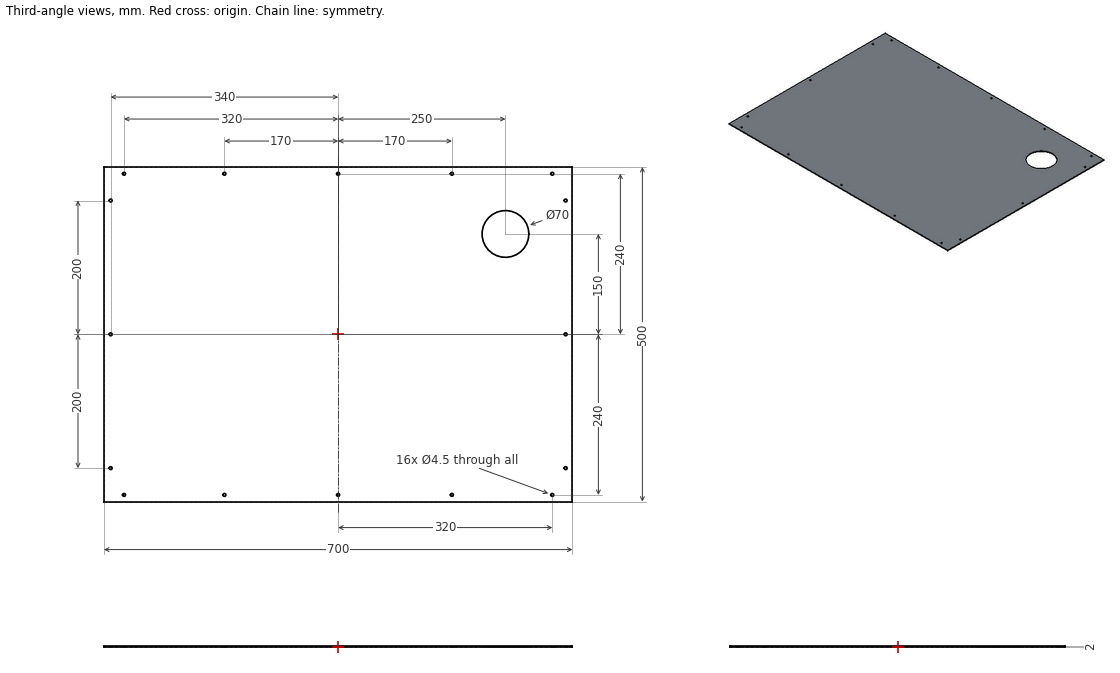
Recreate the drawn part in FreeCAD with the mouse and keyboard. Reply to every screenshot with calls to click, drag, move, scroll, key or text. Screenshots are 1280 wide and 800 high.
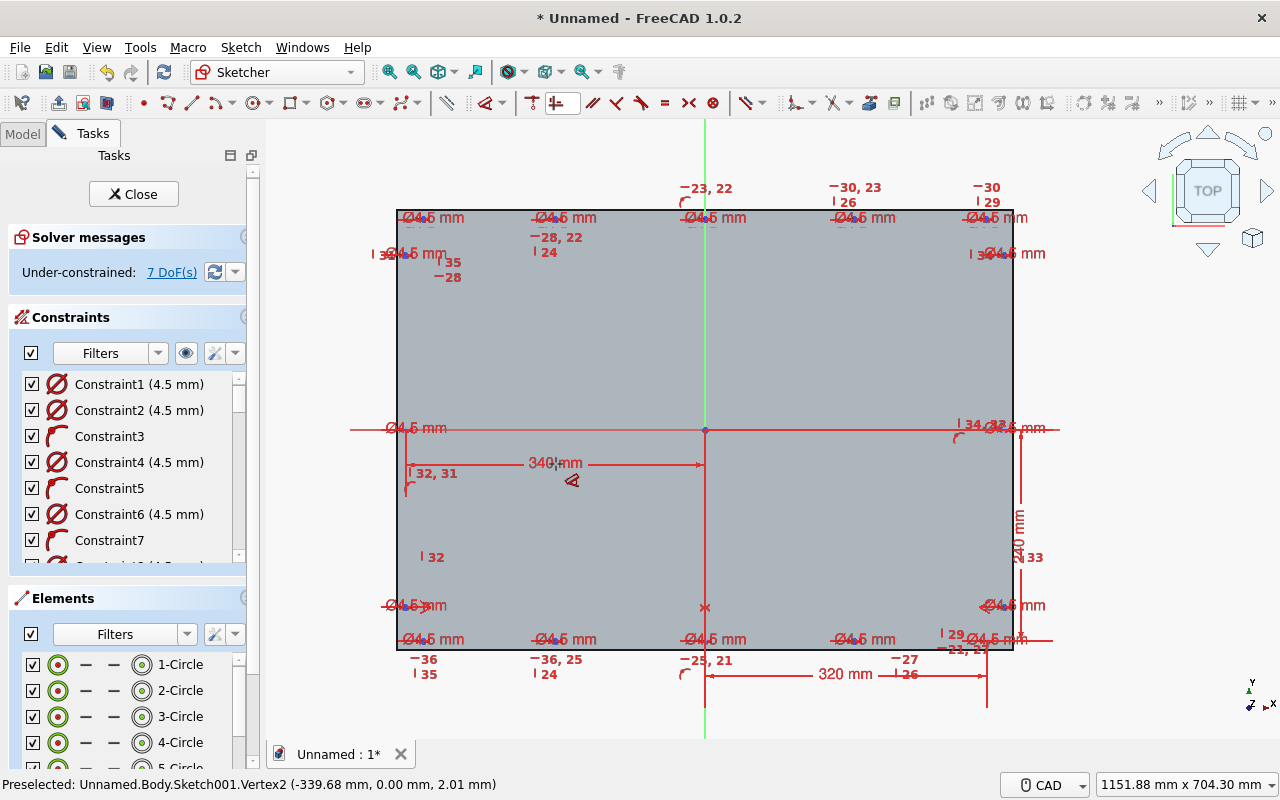
click(705, 220)
click(739, 325)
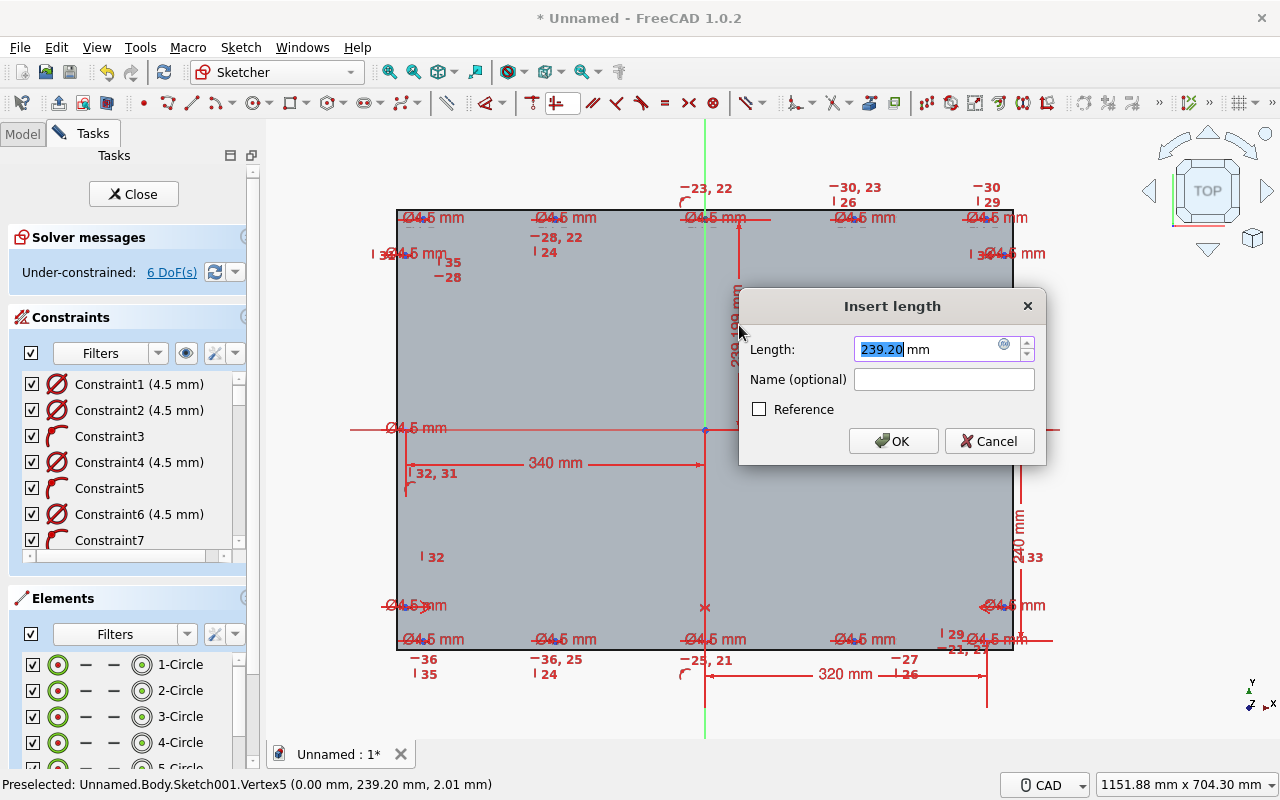
text(240)
key(Return)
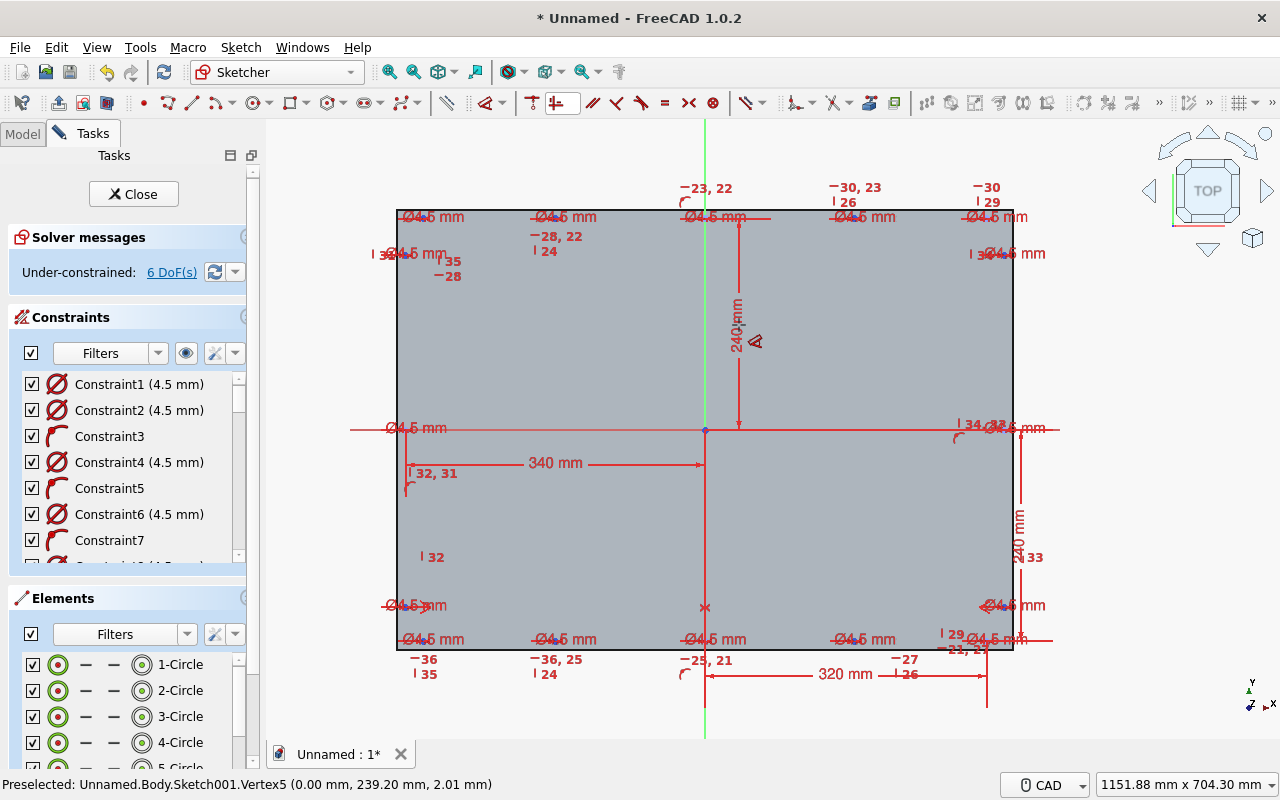
click(556, 219)
click(630, 185)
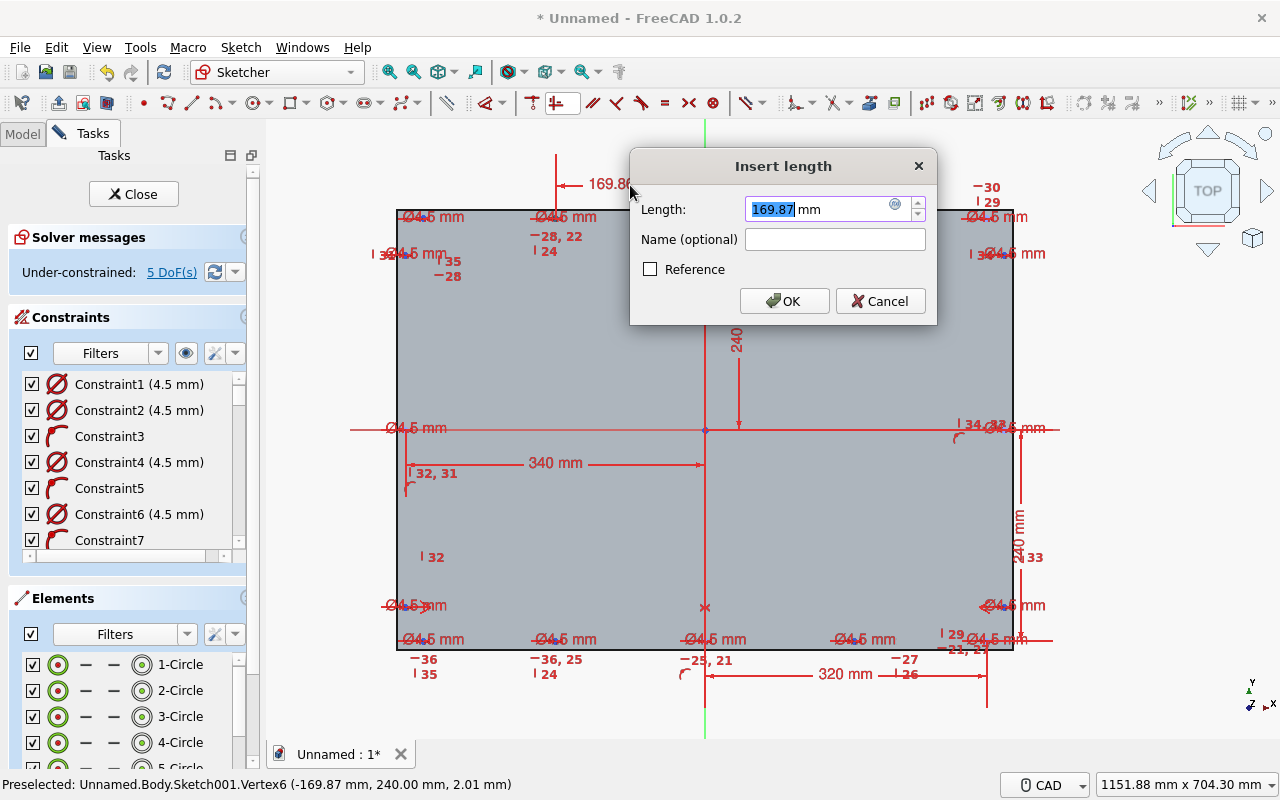
text(170)
key(Return)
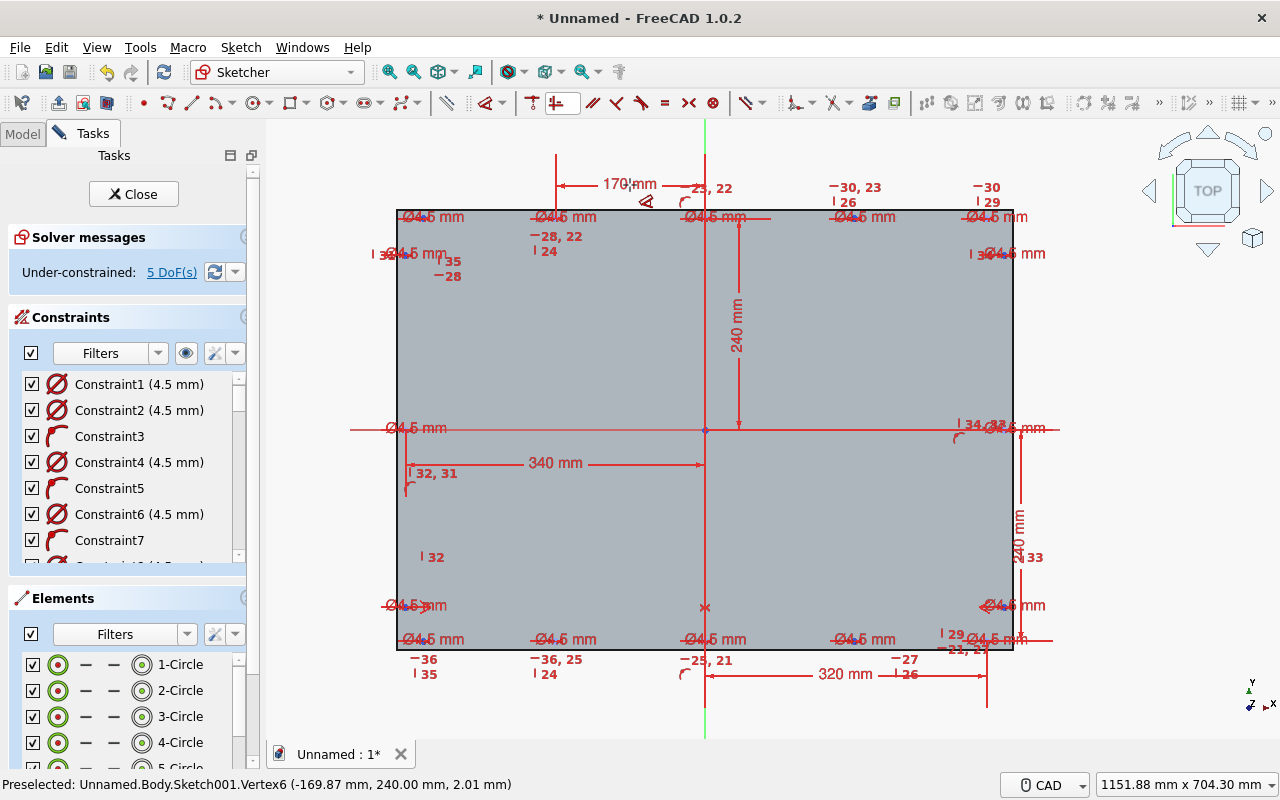
click(855, 219)
click(780, 185)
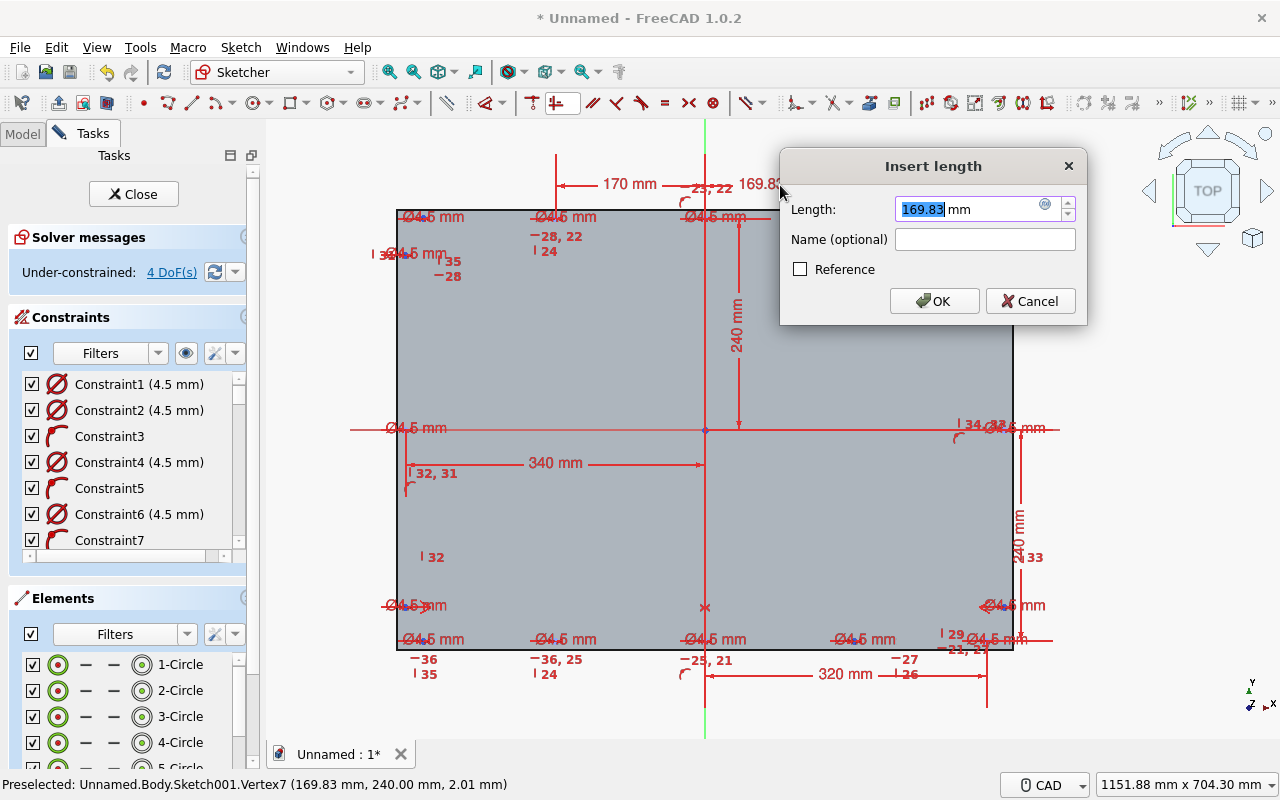
text(170)
key(Return)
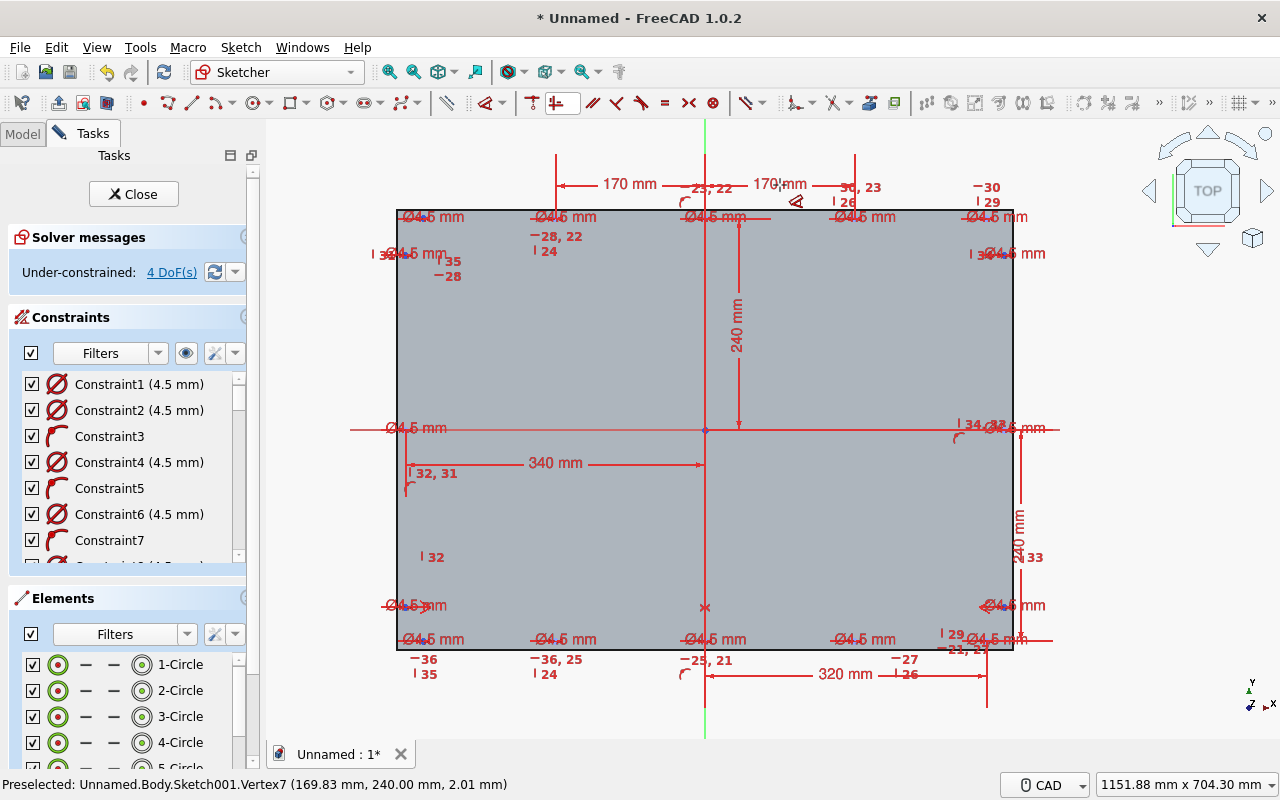
click(423, 219)
click(499, 185)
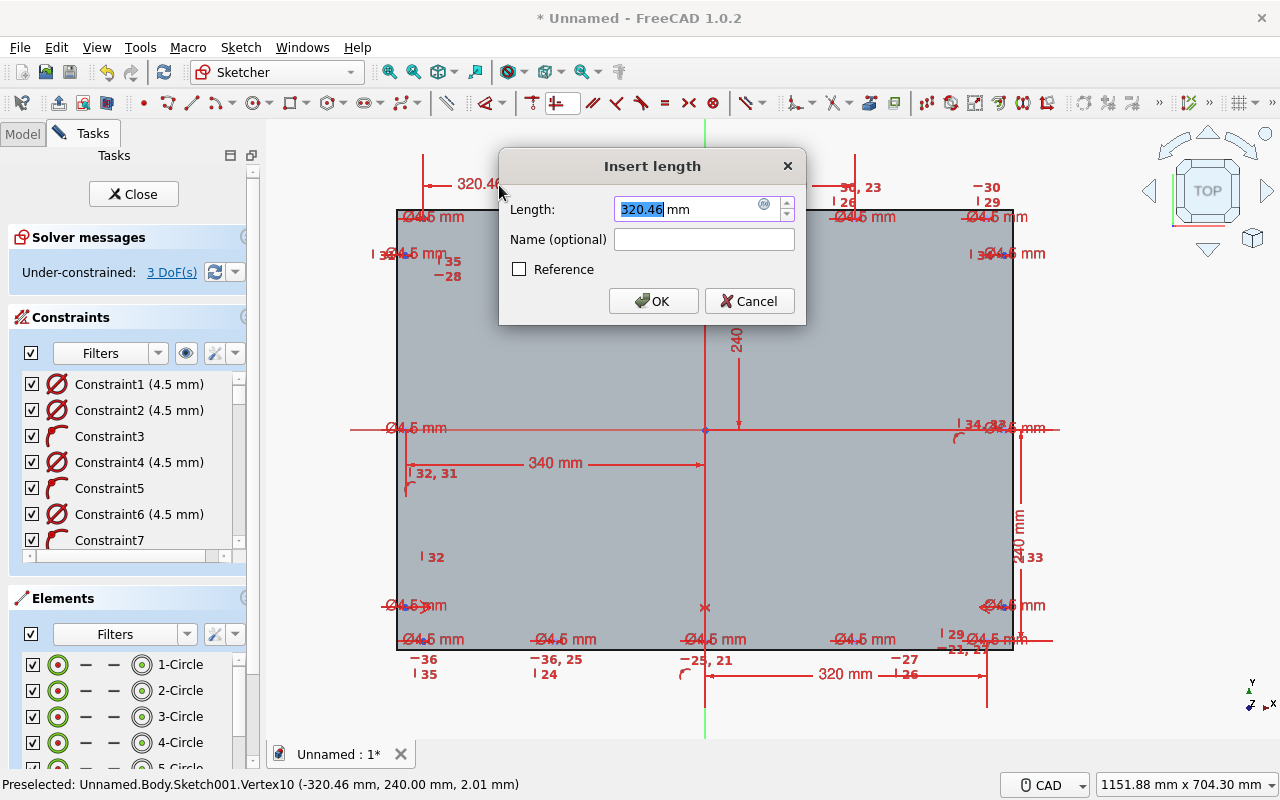
text(320)
key(Return)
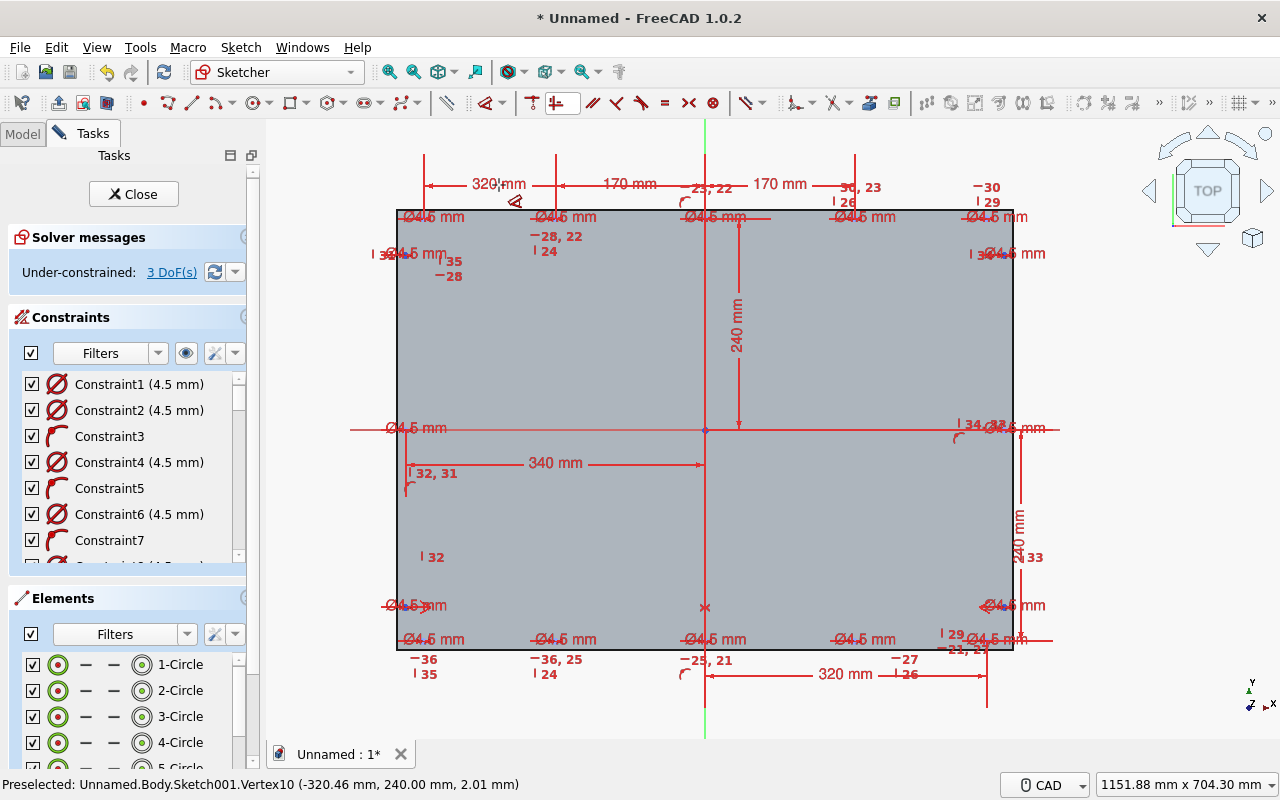
click(406, 255)
click(372, 343)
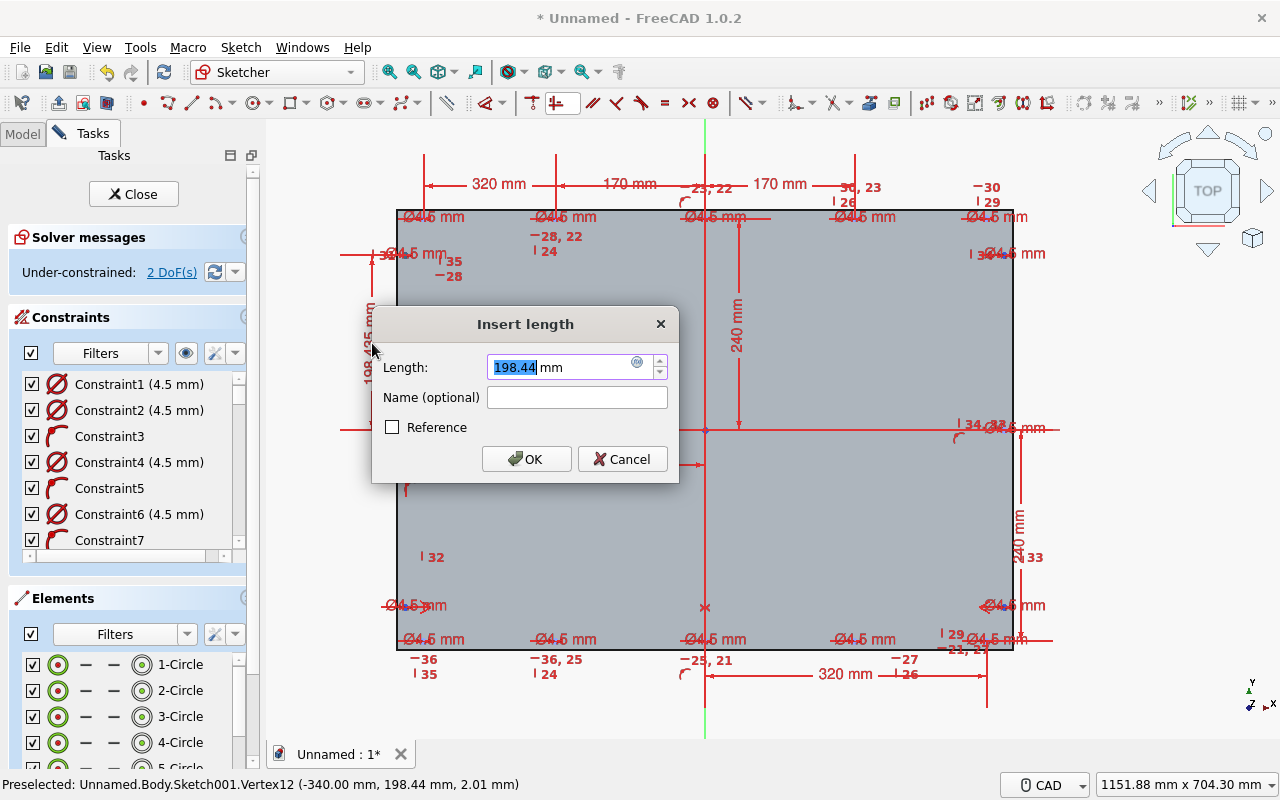
text(200)
key(Return)